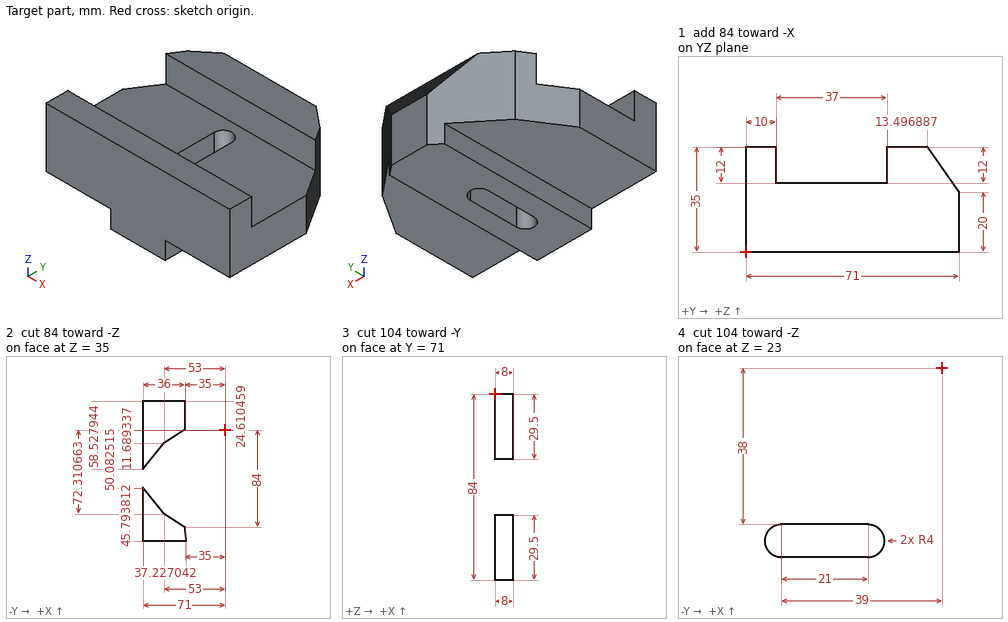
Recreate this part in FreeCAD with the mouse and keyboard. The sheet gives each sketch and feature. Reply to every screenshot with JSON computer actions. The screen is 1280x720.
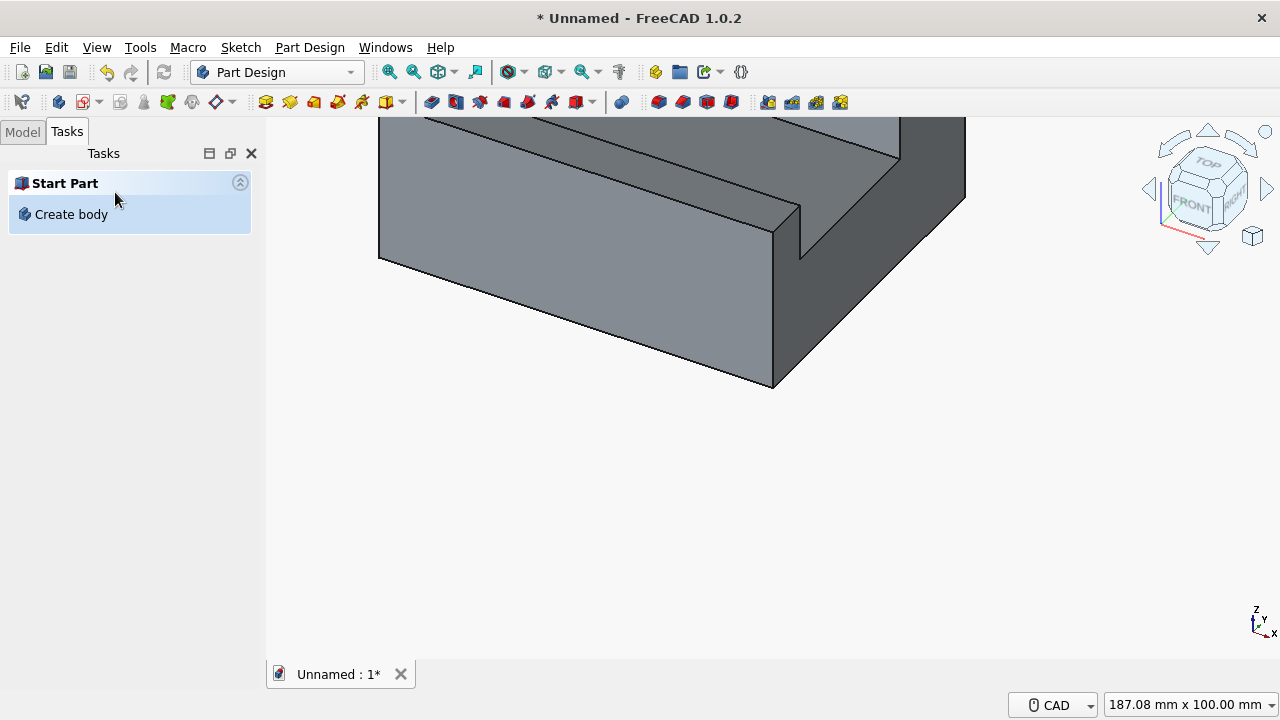
{"action": "left_click", "coordinate": [390, 72]}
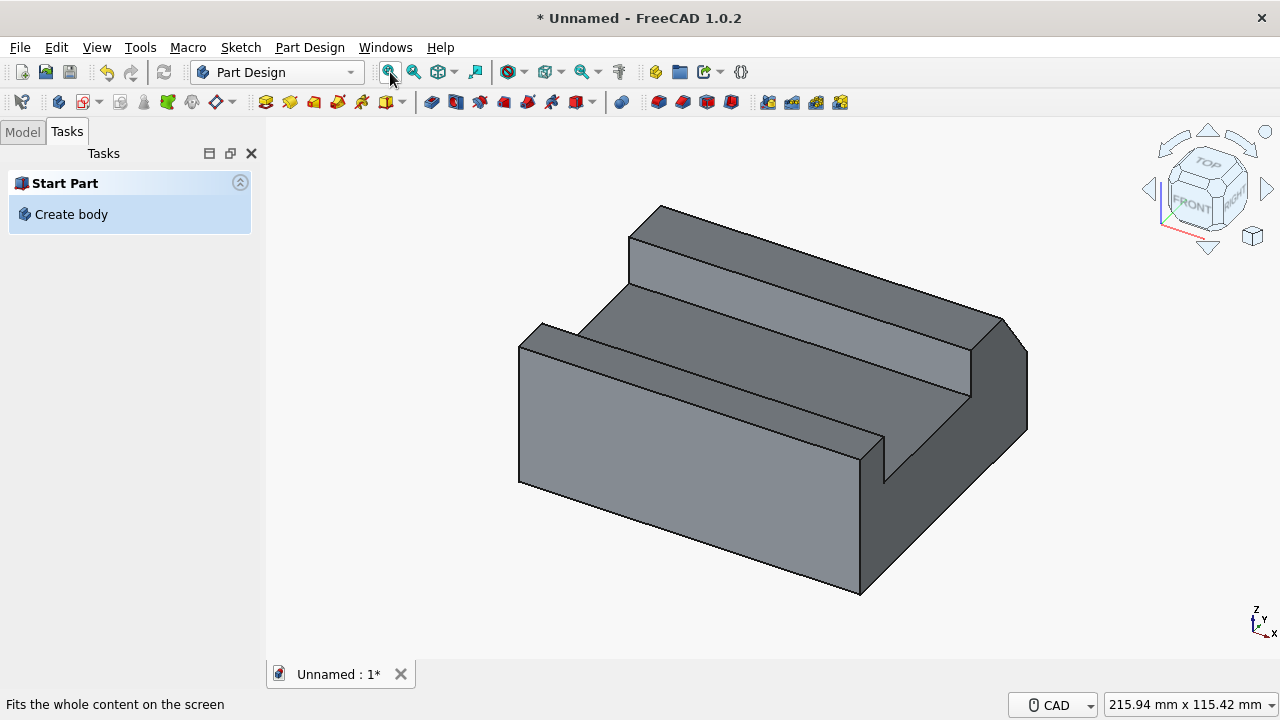
{"action": "left_click", "coordinate": [913, 309]}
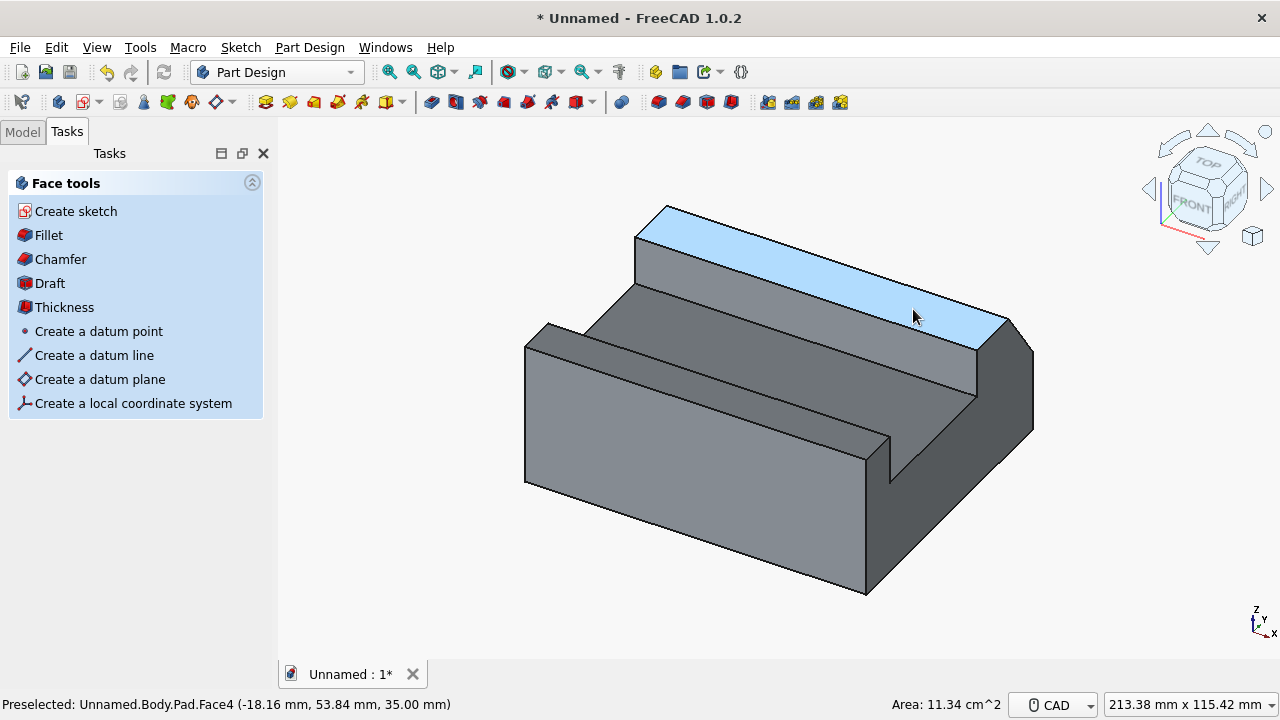
{"action": "left_click", "coordinate": [84, 102]}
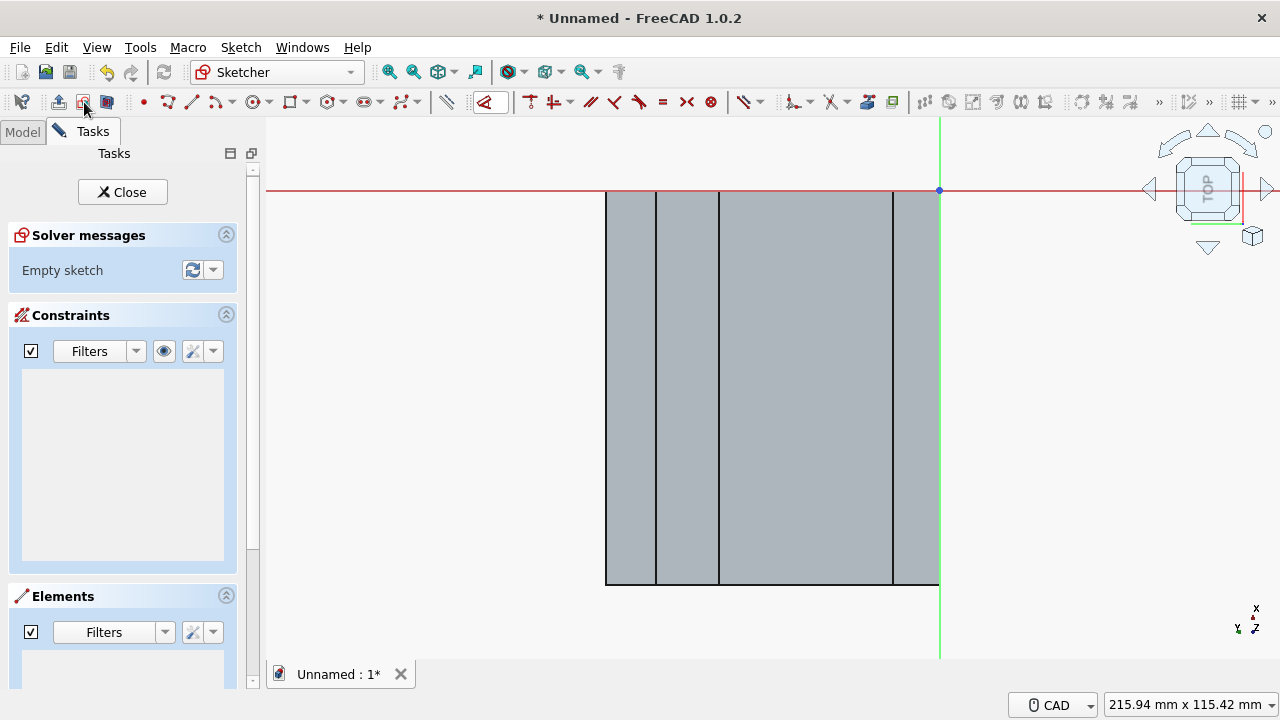
{"action": "scroll", "coordinate": [621, 424], "scroll_direction": "down", "scroll_amount": 3}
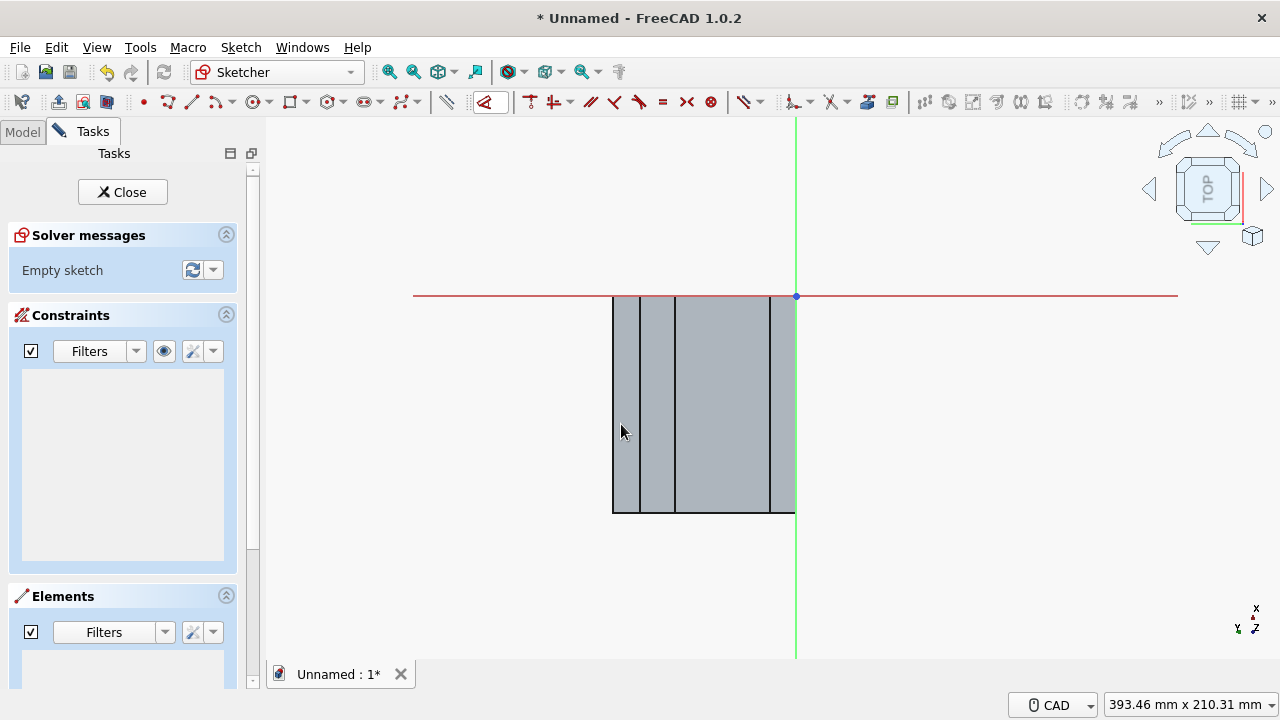
{"action": "left_click", "coordinate": [168, 102]}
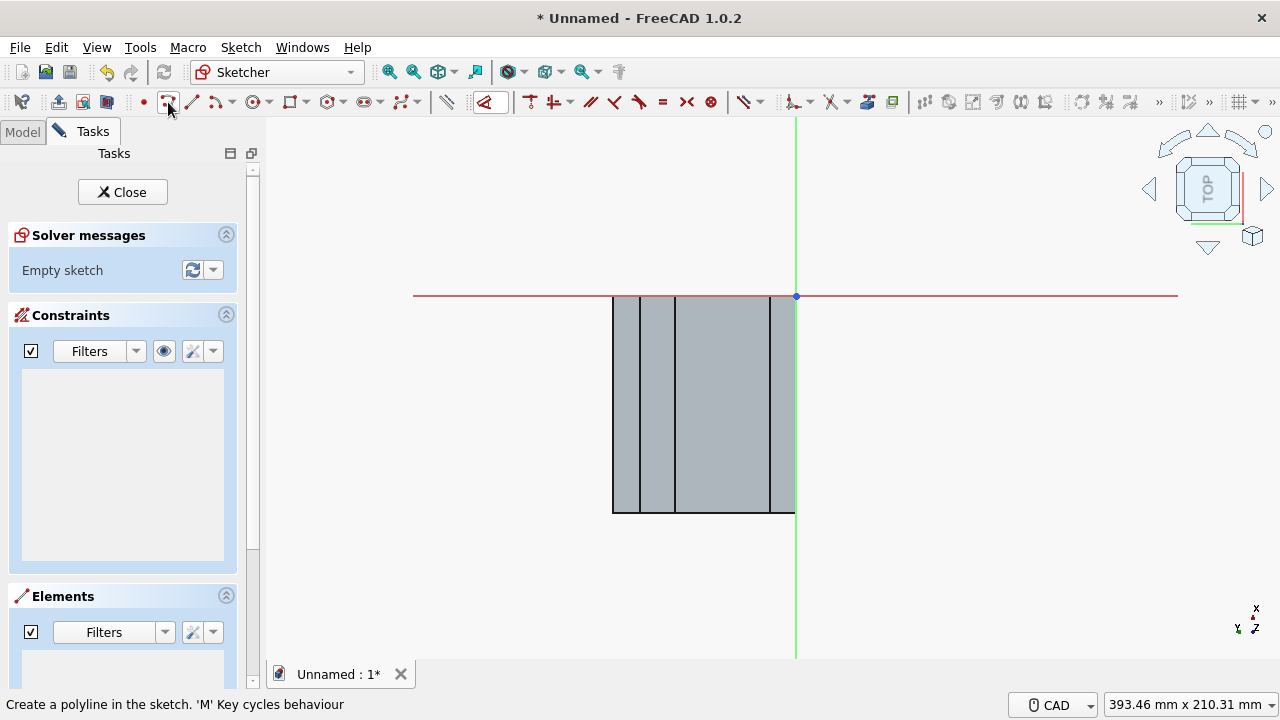
{"action": "left_click", "coordinate": [706, 296]}
{"action": "left_click", "coordinate": [706, 233]}
{"action": "left_click", "coordinate": [613, 233]}
{"action": "left_click", "coordinate": [613, 384]}
{"action": "left_click", "coordinate": [659, 326]}
{"action": "left_click", "coordinate": [706, 296]}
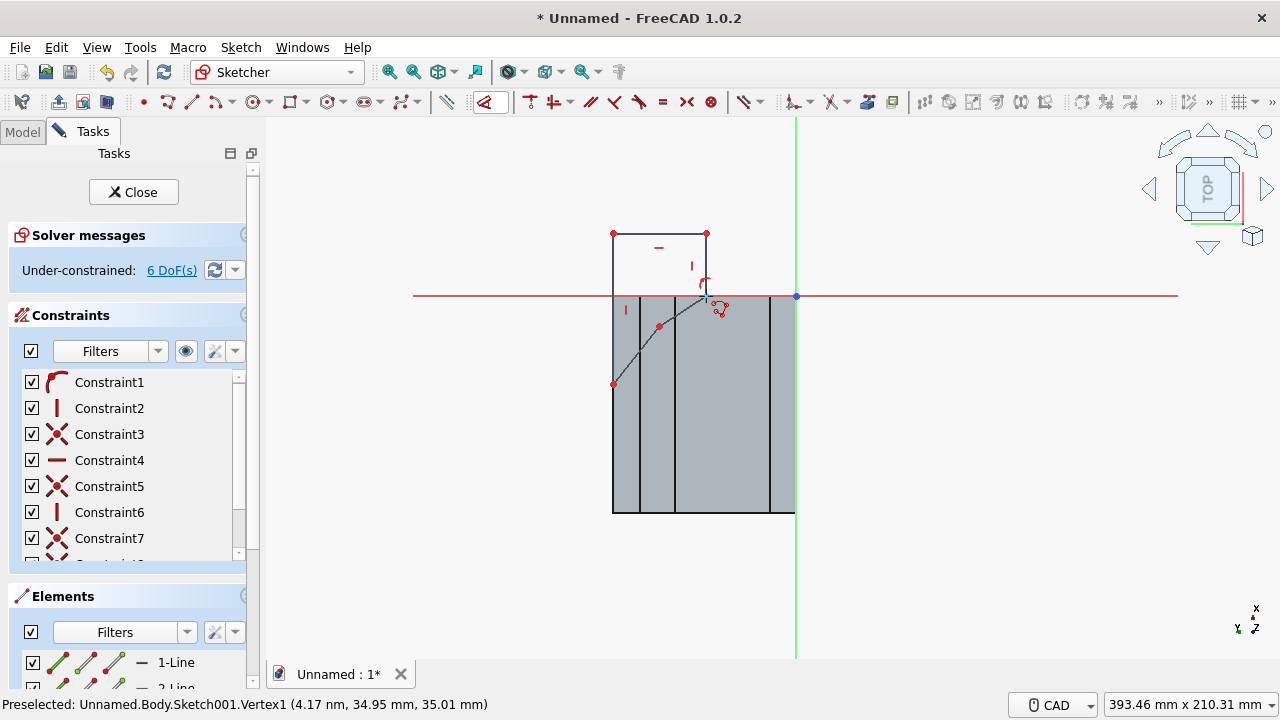
{"action": "left_click", "coordinate": [613, 425]}
{"action": "left_click", "coordinate": [613, 543]}
{"action": "left_click", "coordinate": [709, 543]}
{"action": "left_click", "coordinate": [706, 513]}
{"action": "left_click", "coordinate": [659, 483]}
{"action": "left_click", "coordinate": [613, 426]}
{"action": "key", "text": "Escape"}
{"action": "key", "text": "Escape"}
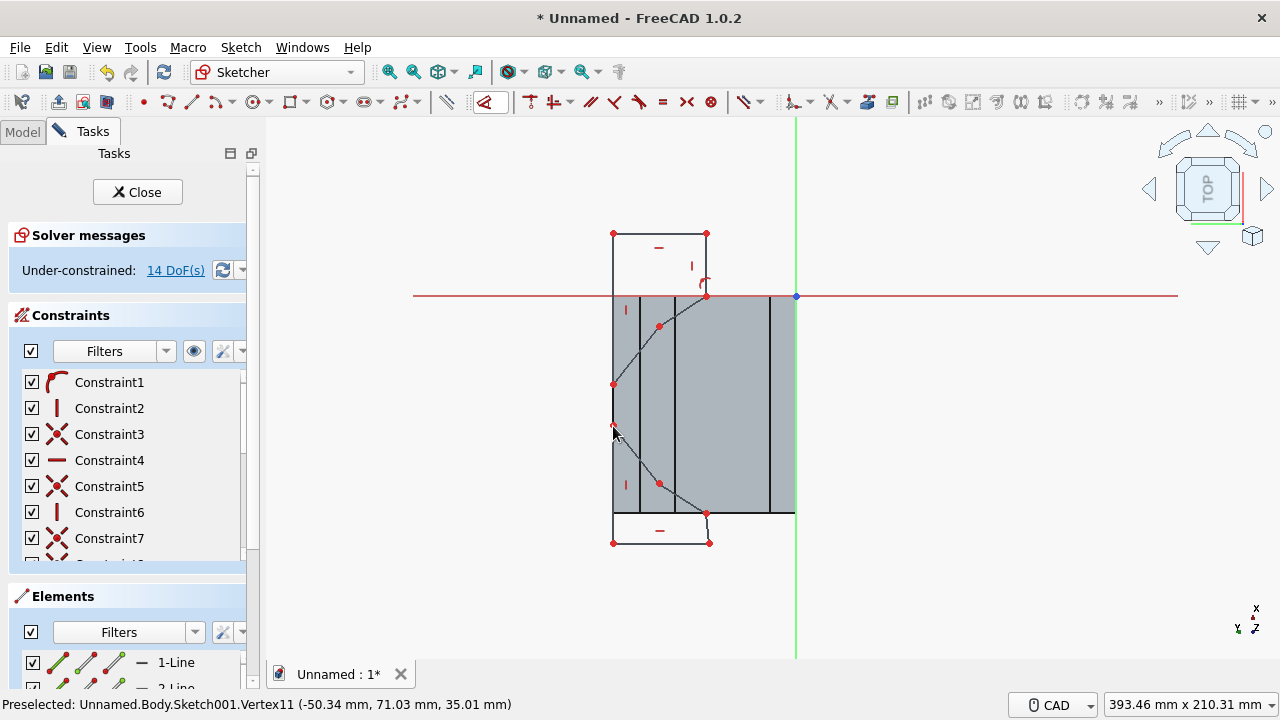
{"action": "left_click", "coordinate": [678, 234]}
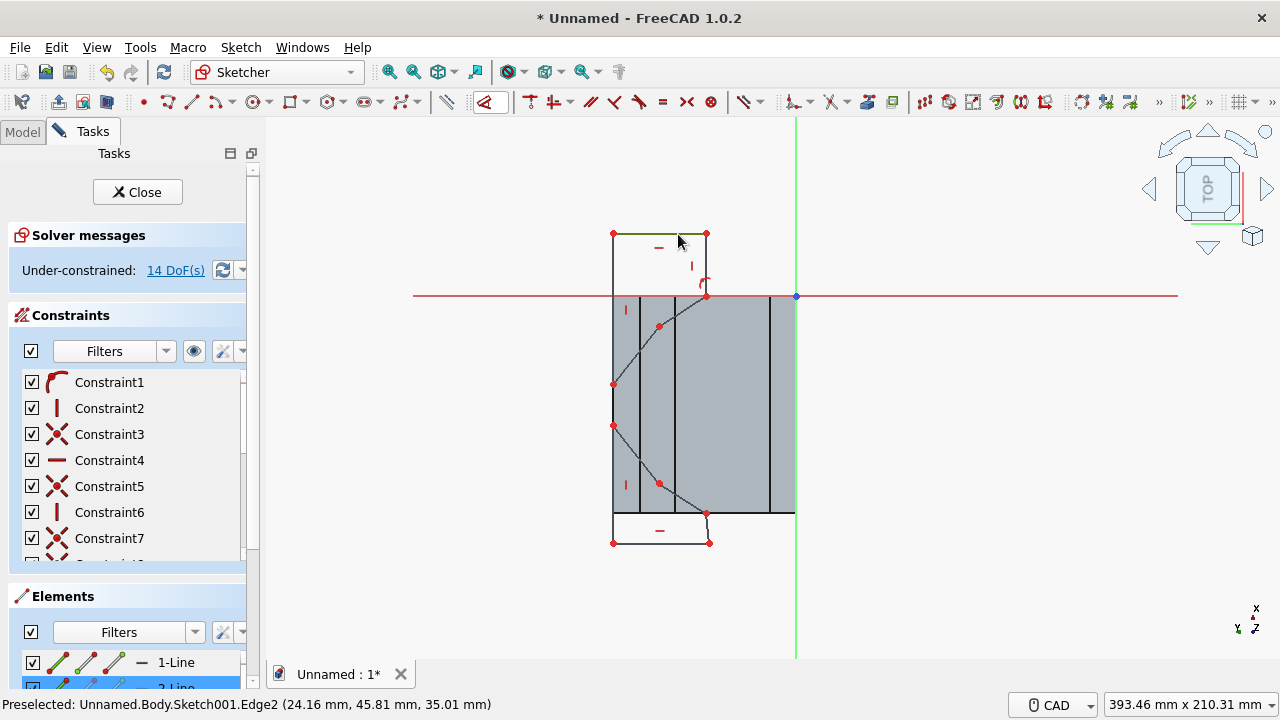
{"action": "left_click", "coordinate": [502, 102]}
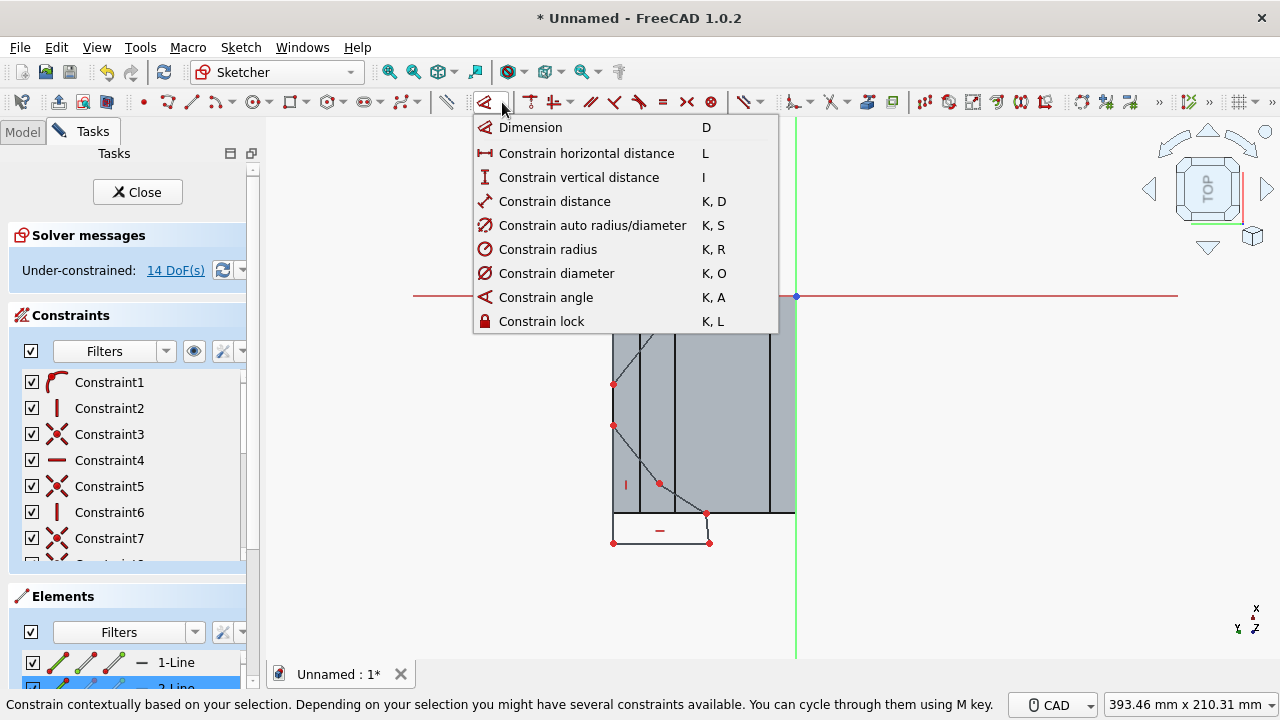
{"action": "left_click", "coordinate": [626, 153]}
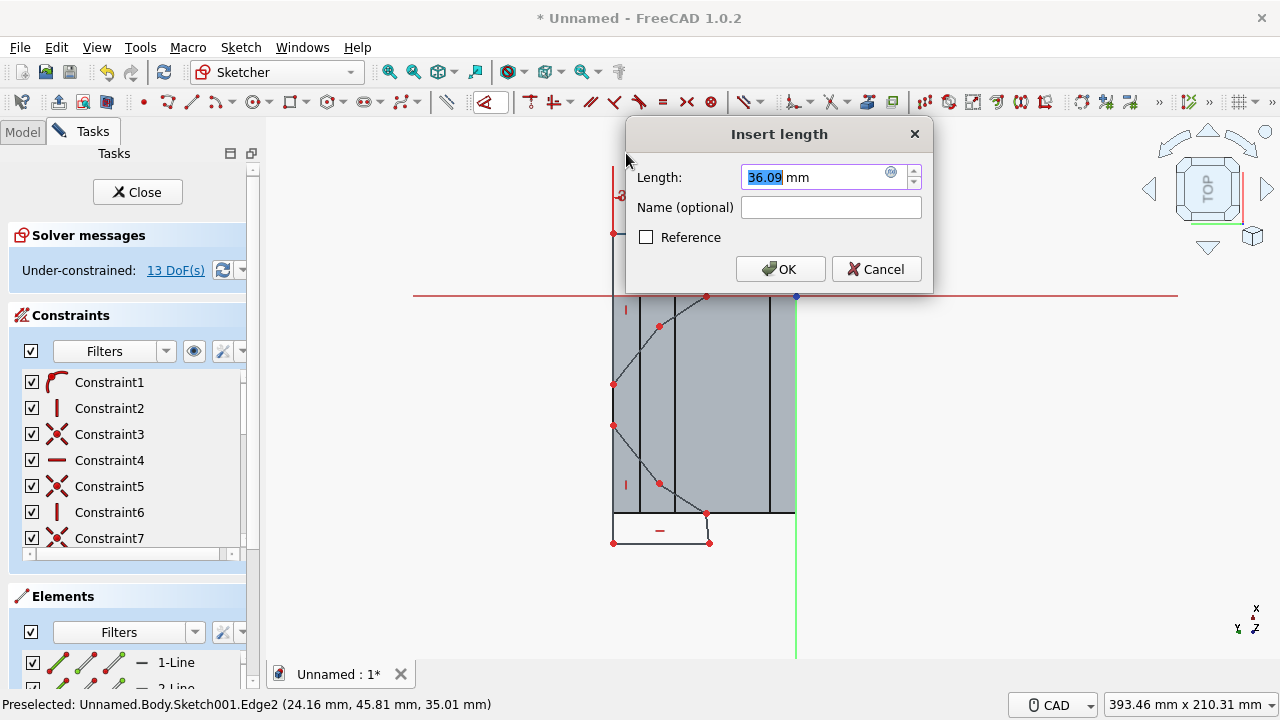
{"action": "type", "text": "36"}
{"action": "key", "text": "Return"}